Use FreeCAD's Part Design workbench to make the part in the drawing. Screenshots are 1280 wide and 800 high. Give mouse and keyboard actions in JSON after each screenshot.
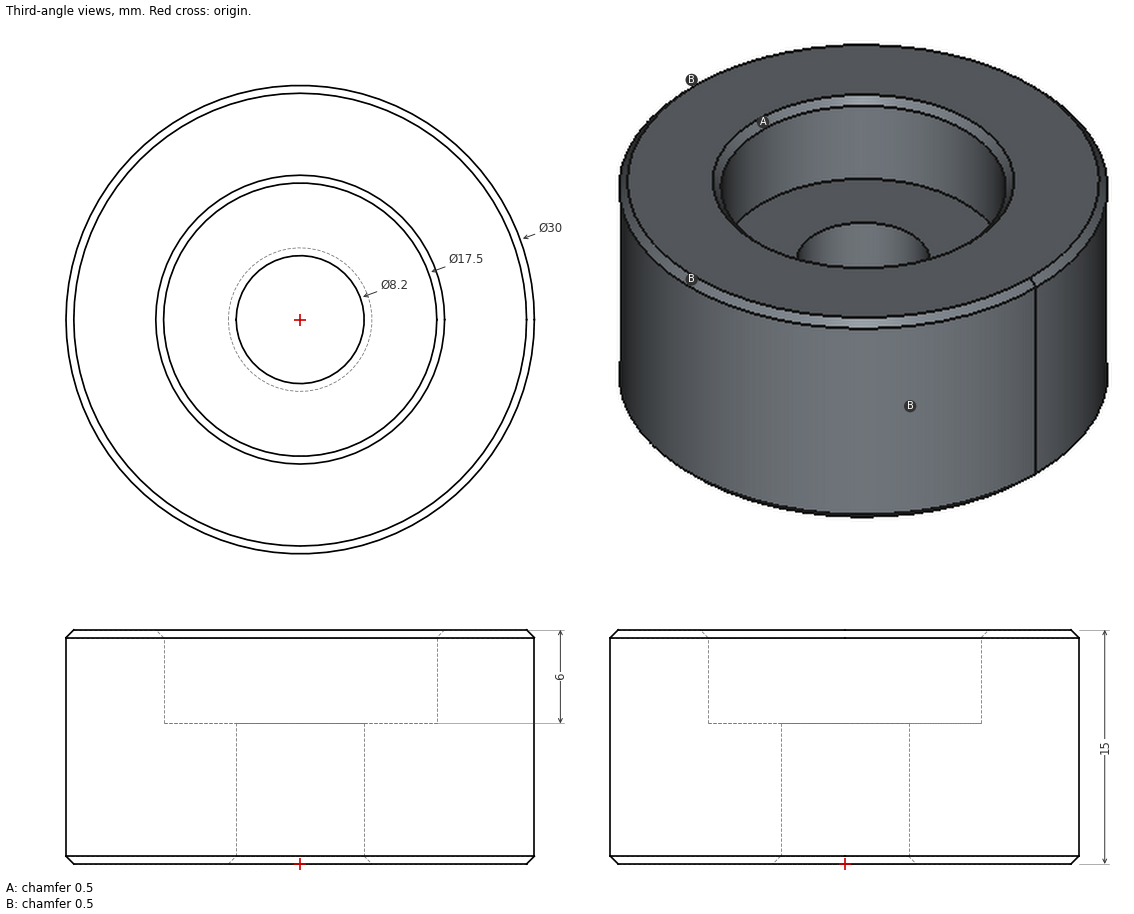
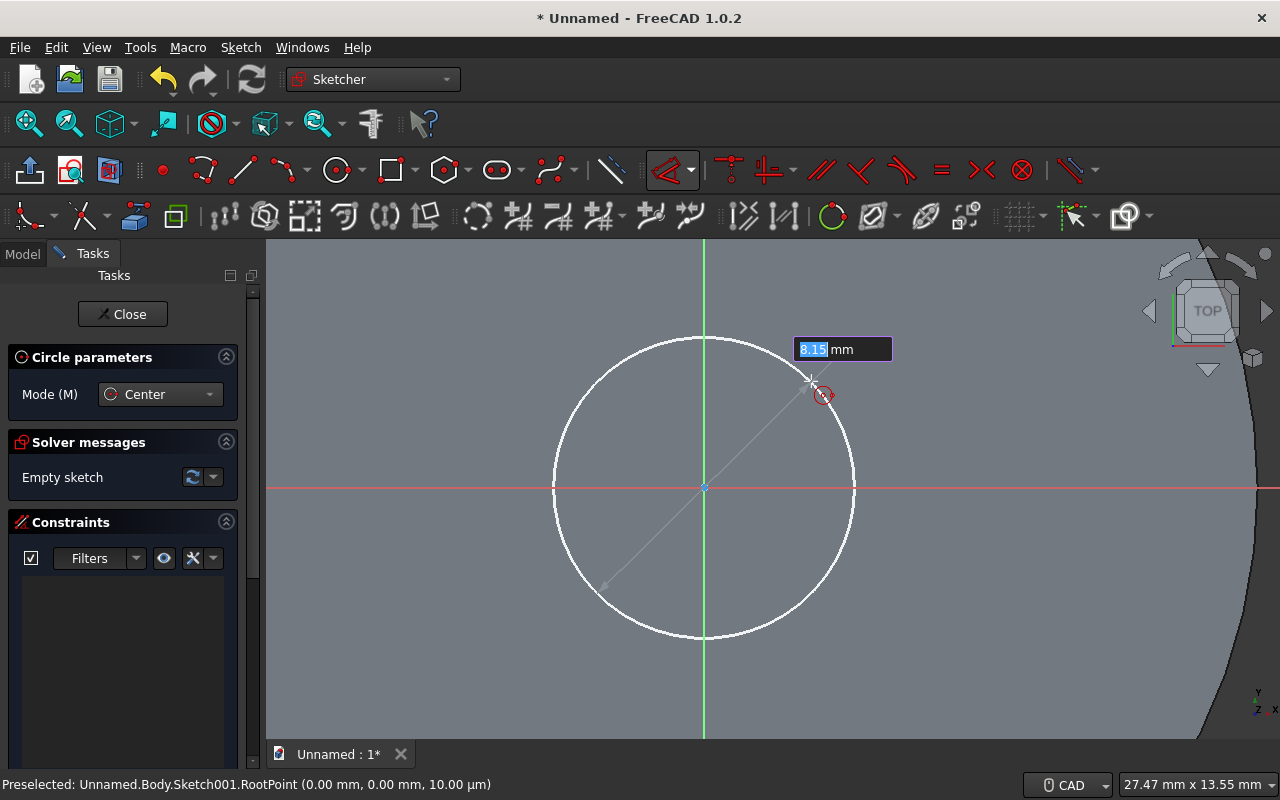
{"action": "type", "text": "8.2"}
{"action": "key", "text": "Return"}
{"action": "key", "text": "Escape"}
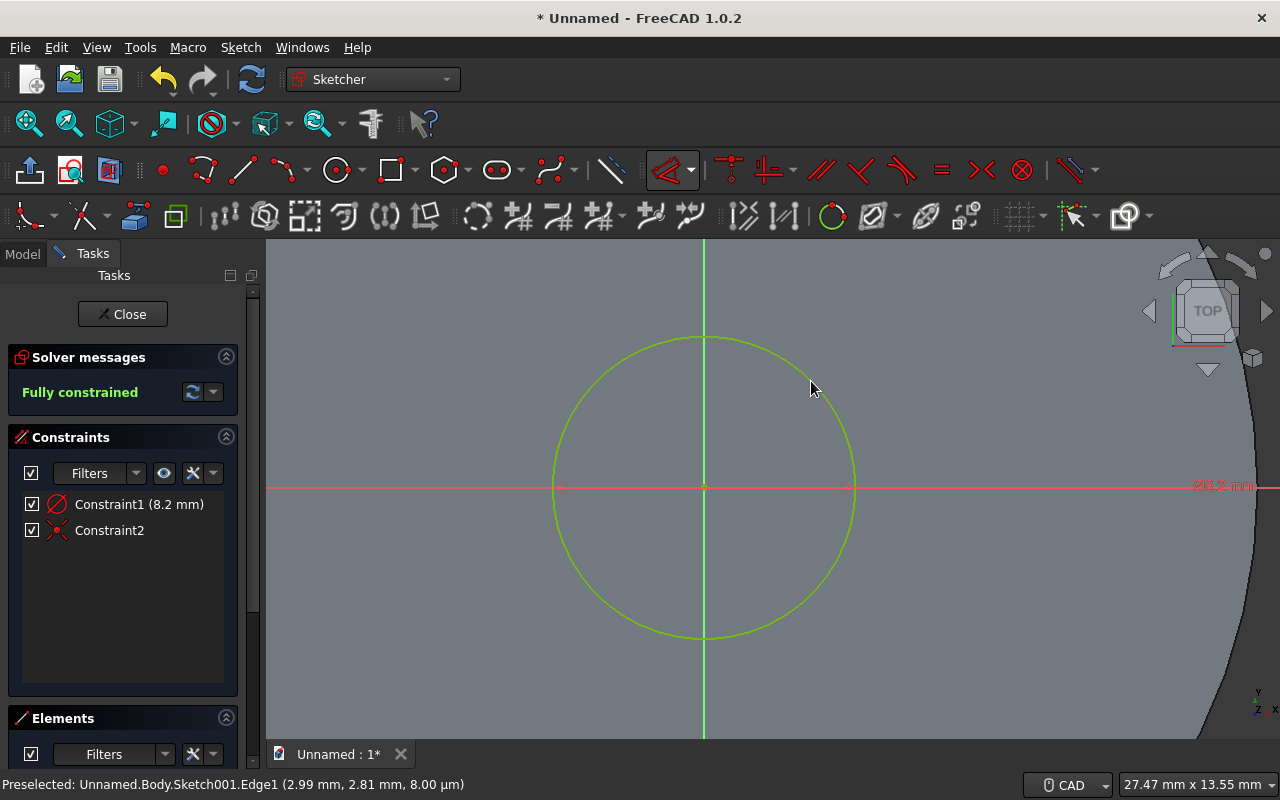
{"action": "left_click", "coordinate": [123, 314]}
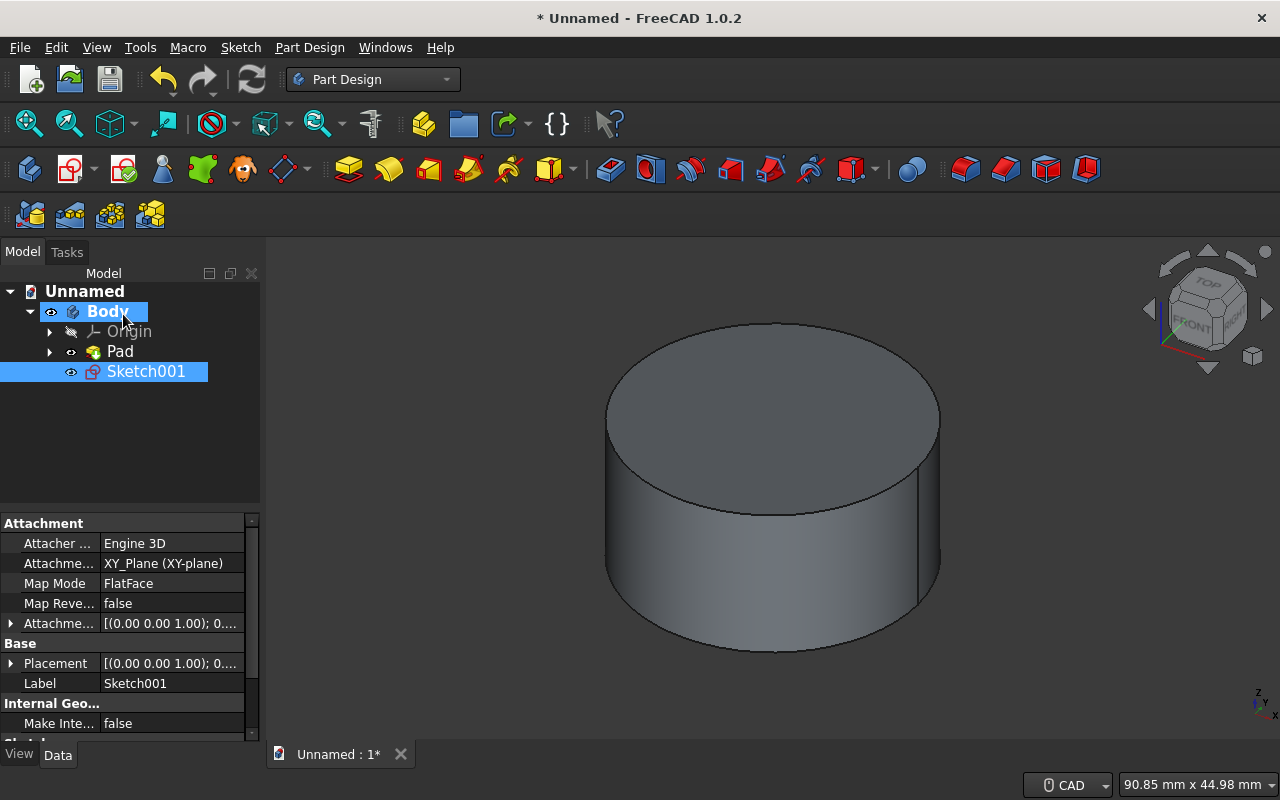
{"action": "left_click", "coordinate": [612, 170]}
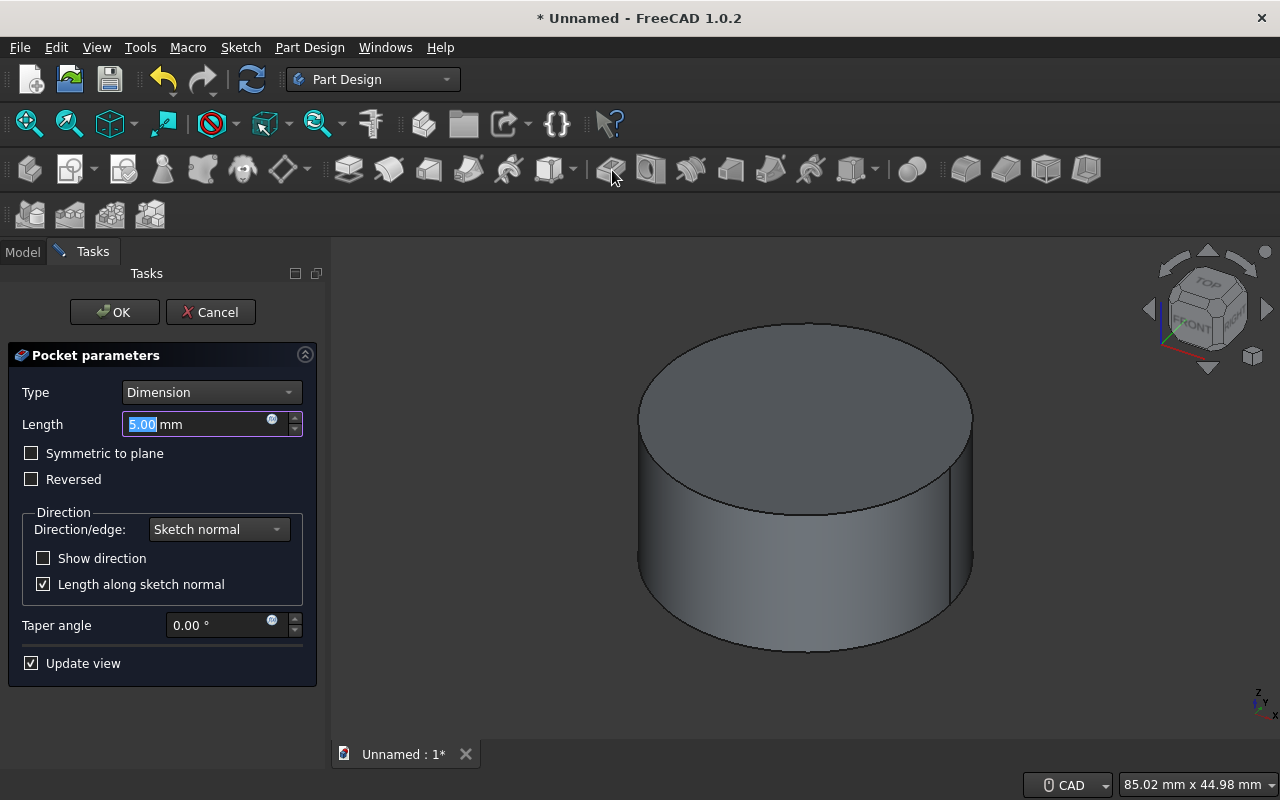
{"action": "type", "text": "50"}
{"action": "key", "text": "Tab"}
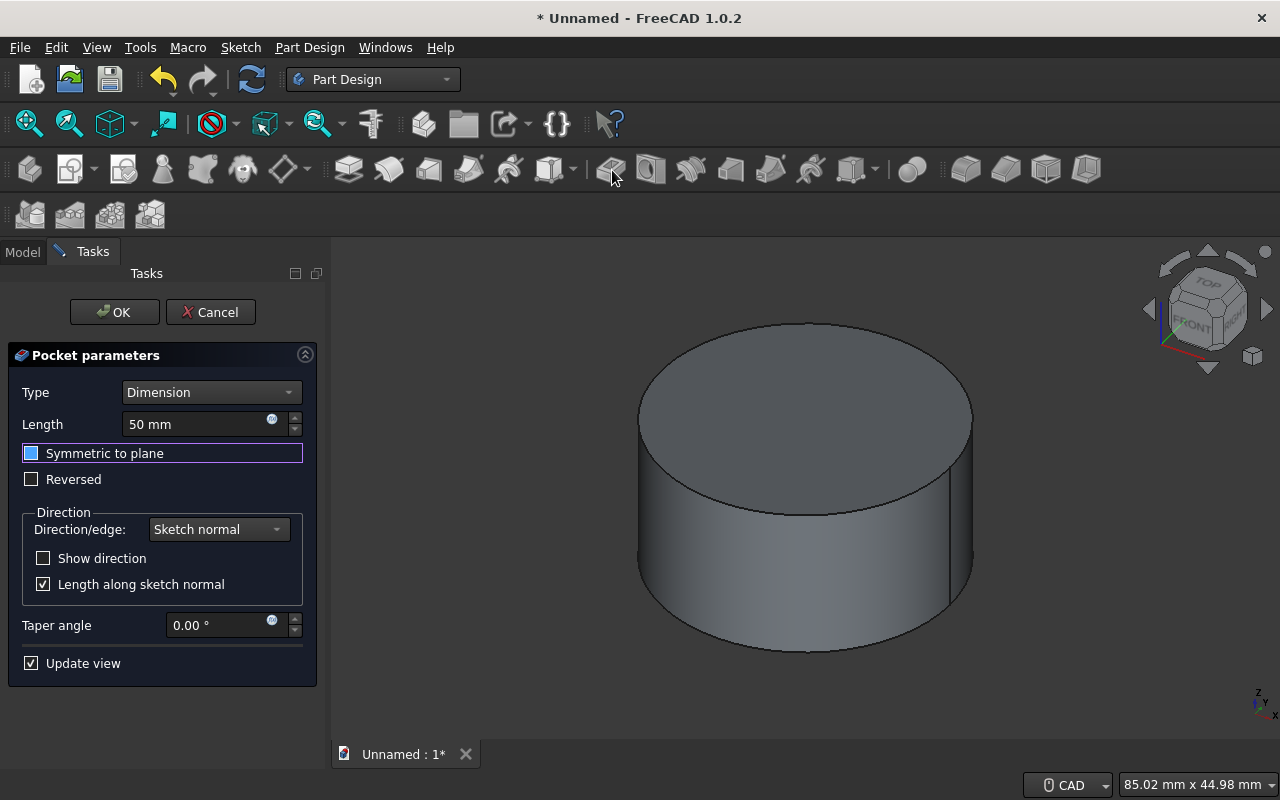
{"action": "left_click", "coordinate": [30, 479]}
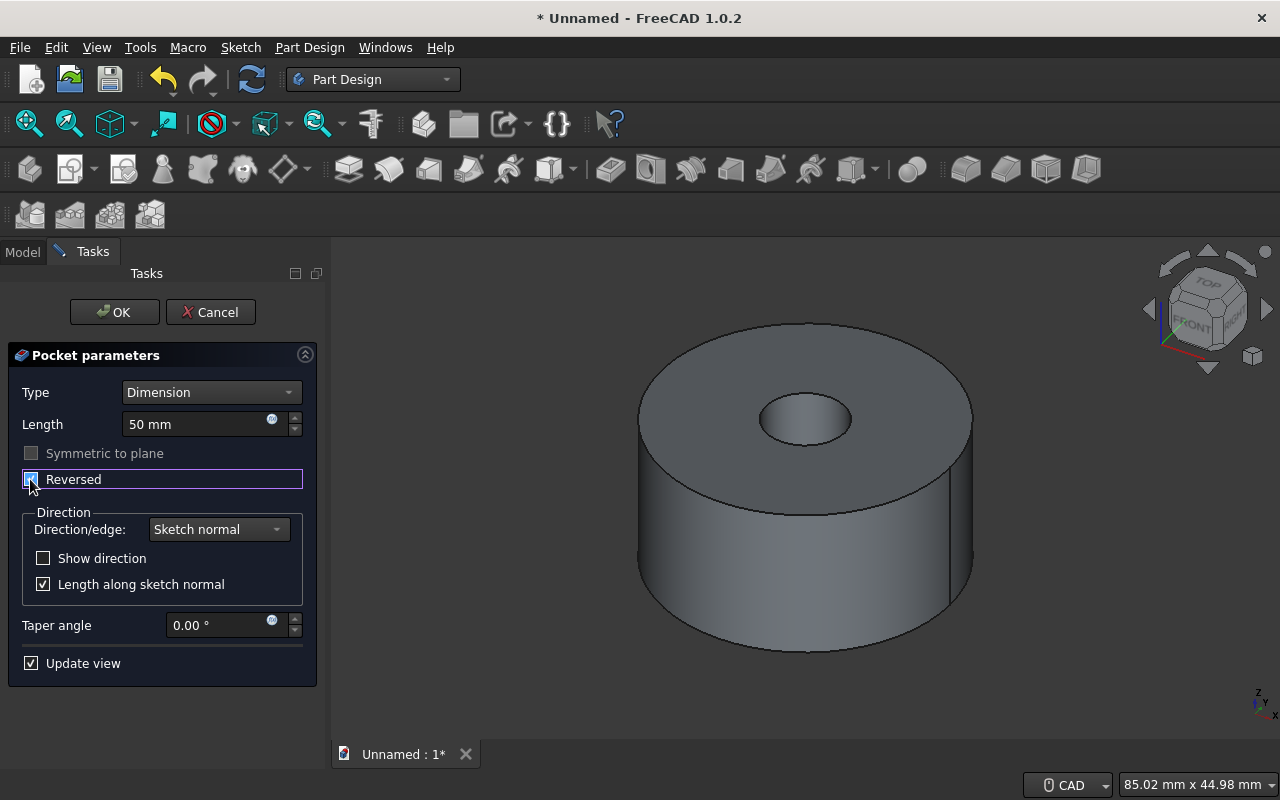
{"action": "left_click", "coordinate": [115, 312]}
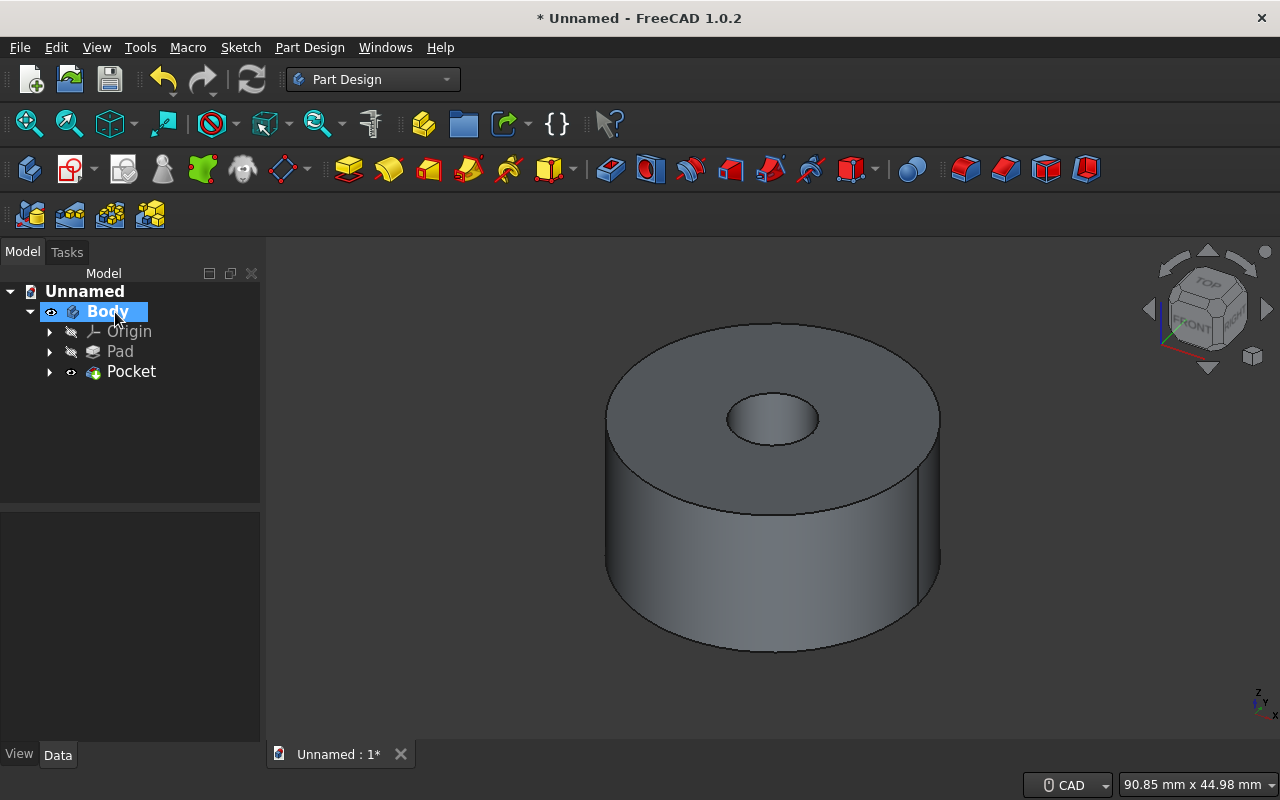
{"action": "left_click", "coordinate": [766, 480]}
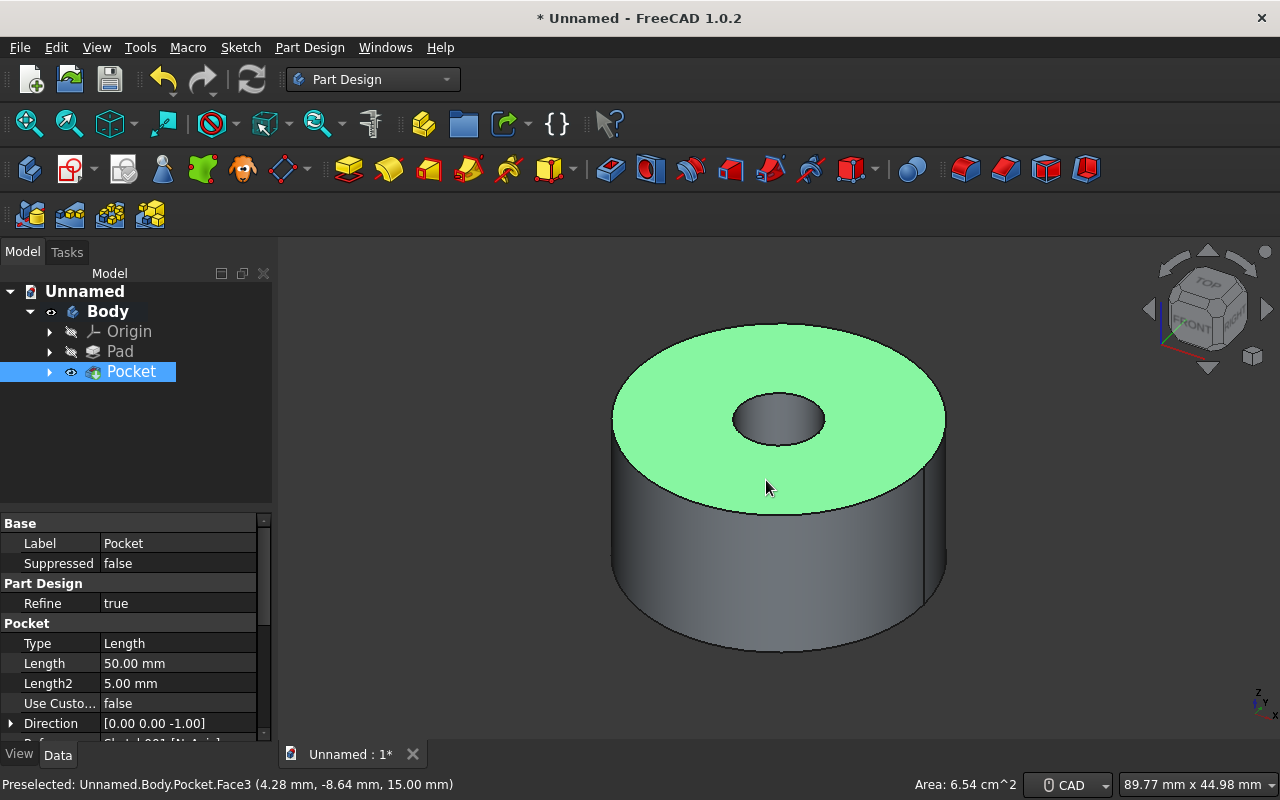
{"action": "left_click", "coordinate": [70, 170]}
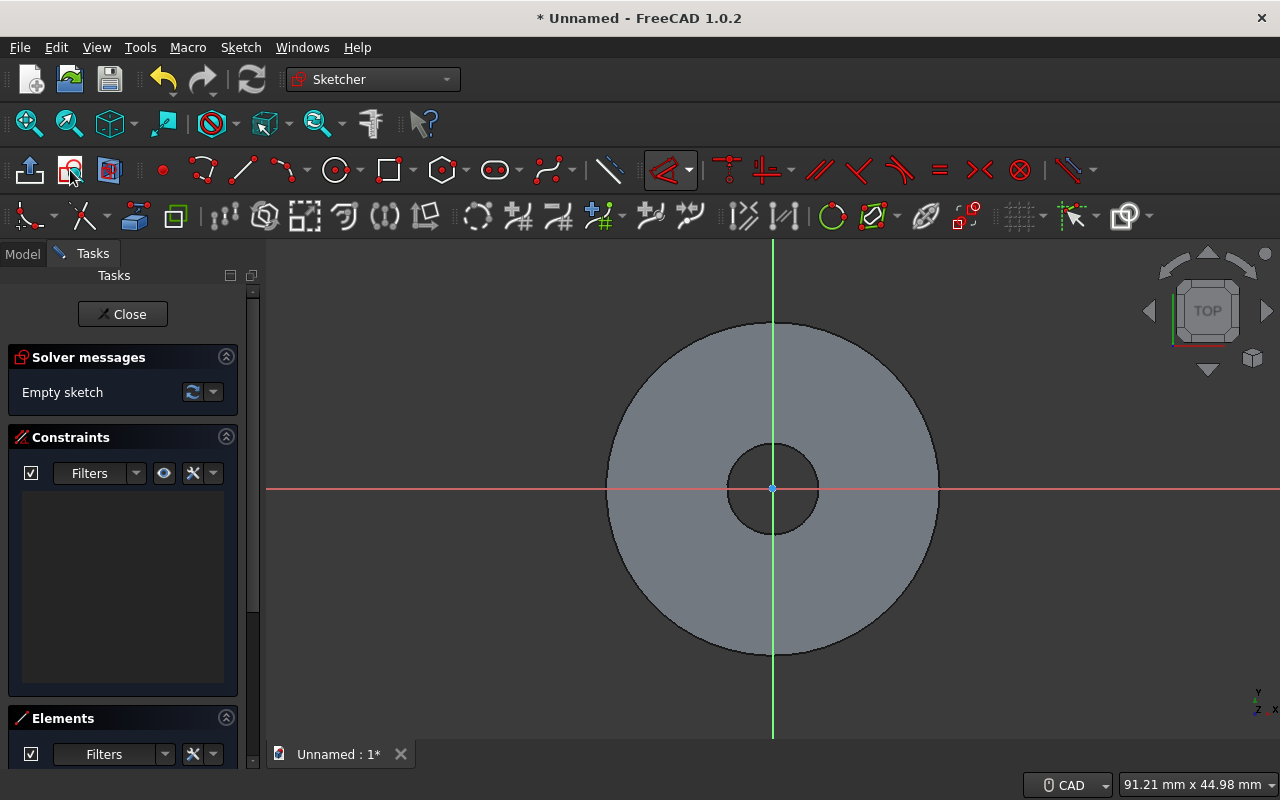
{"action": "scroll", "coordinate": [912, 489], "scroll_direction": "up", "scroll_amount": 2}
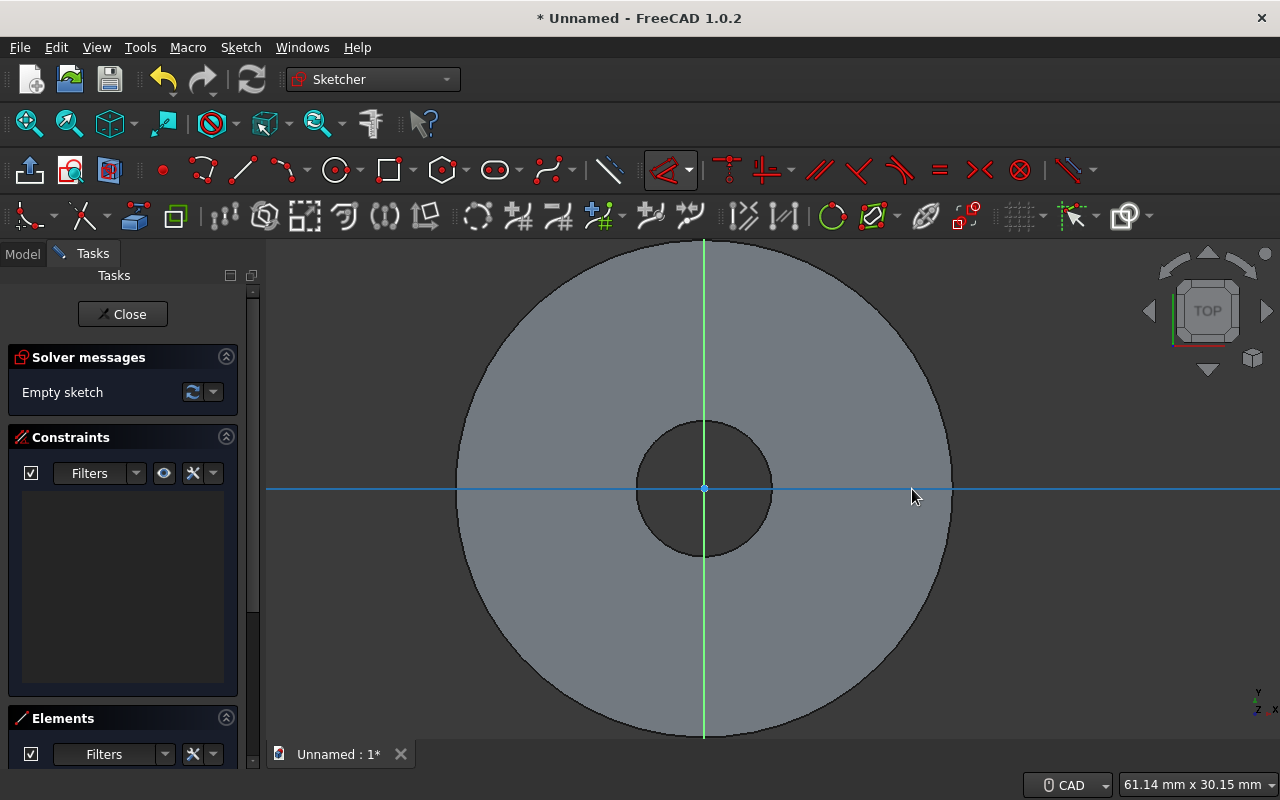
{"action": "left_click", "coordinate": [336, 170]}